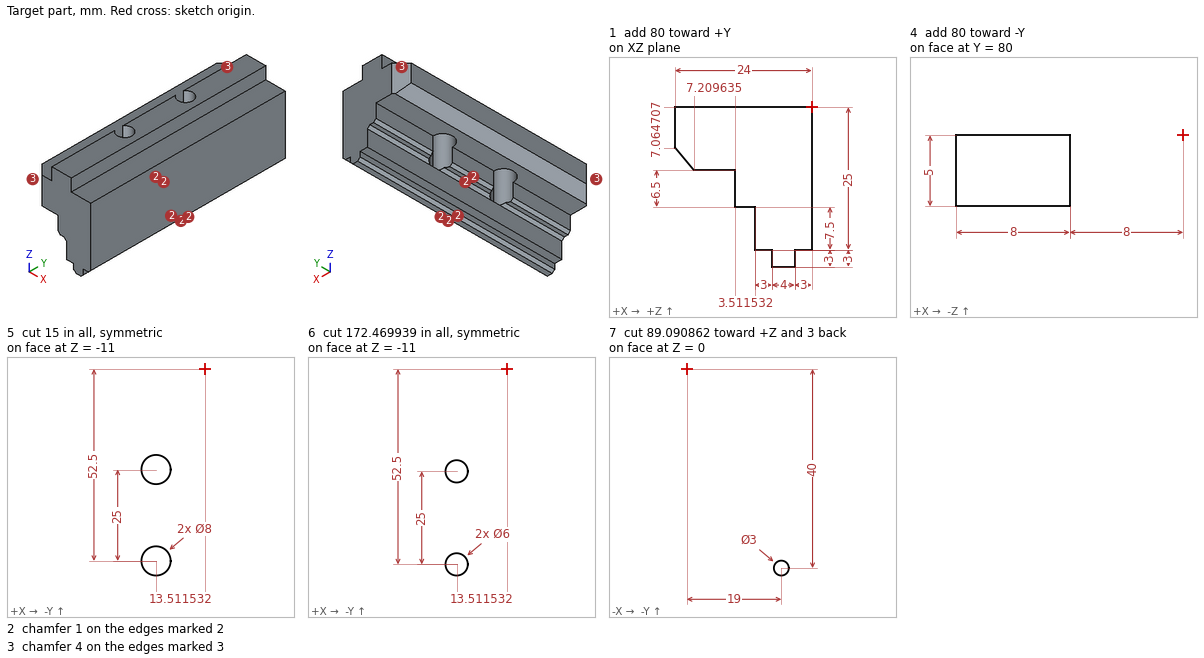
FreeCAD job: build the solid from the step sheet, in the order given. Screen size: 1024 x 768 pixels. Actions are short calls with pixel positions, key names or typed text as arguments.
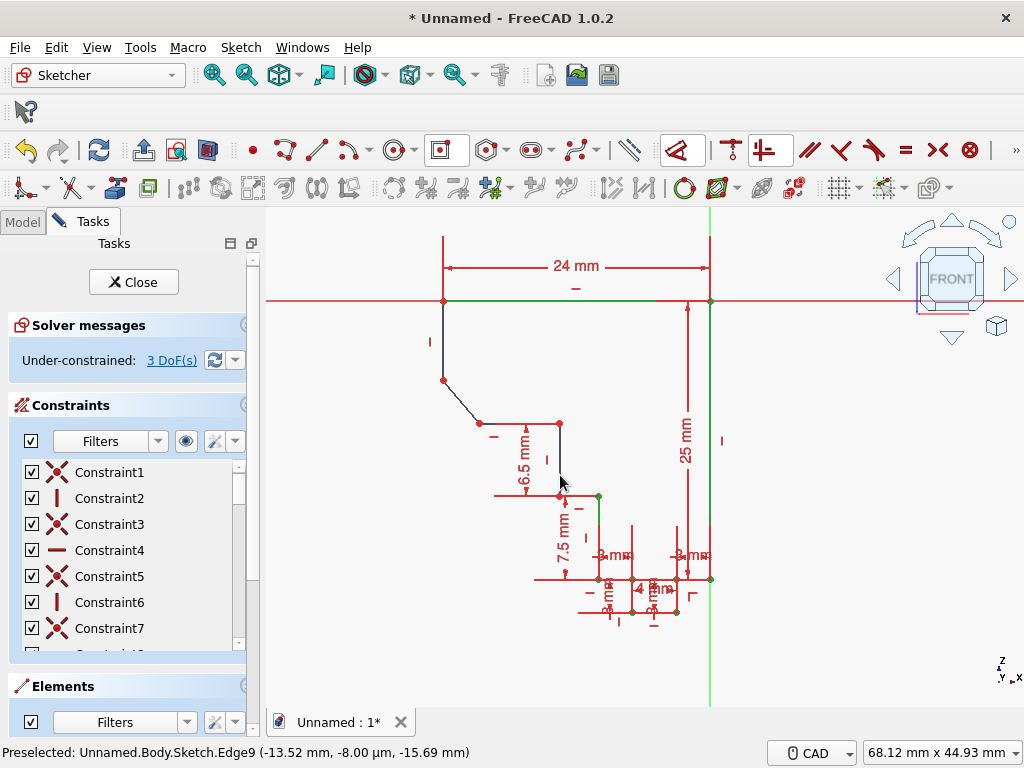
click(587, 496)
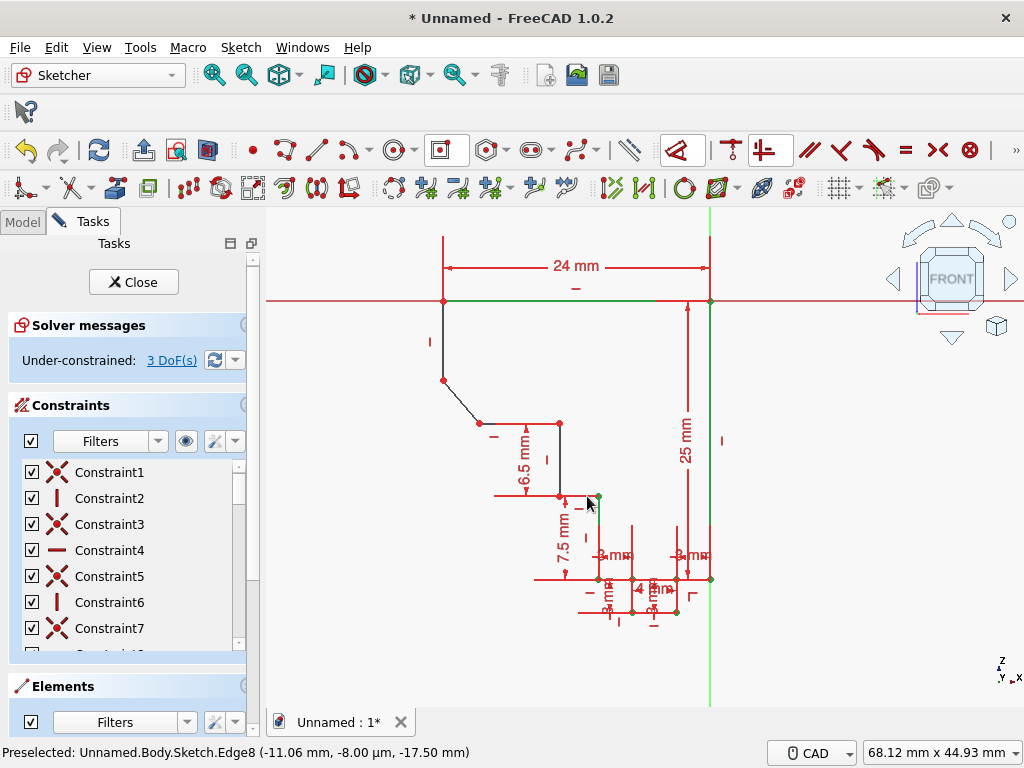
key(l)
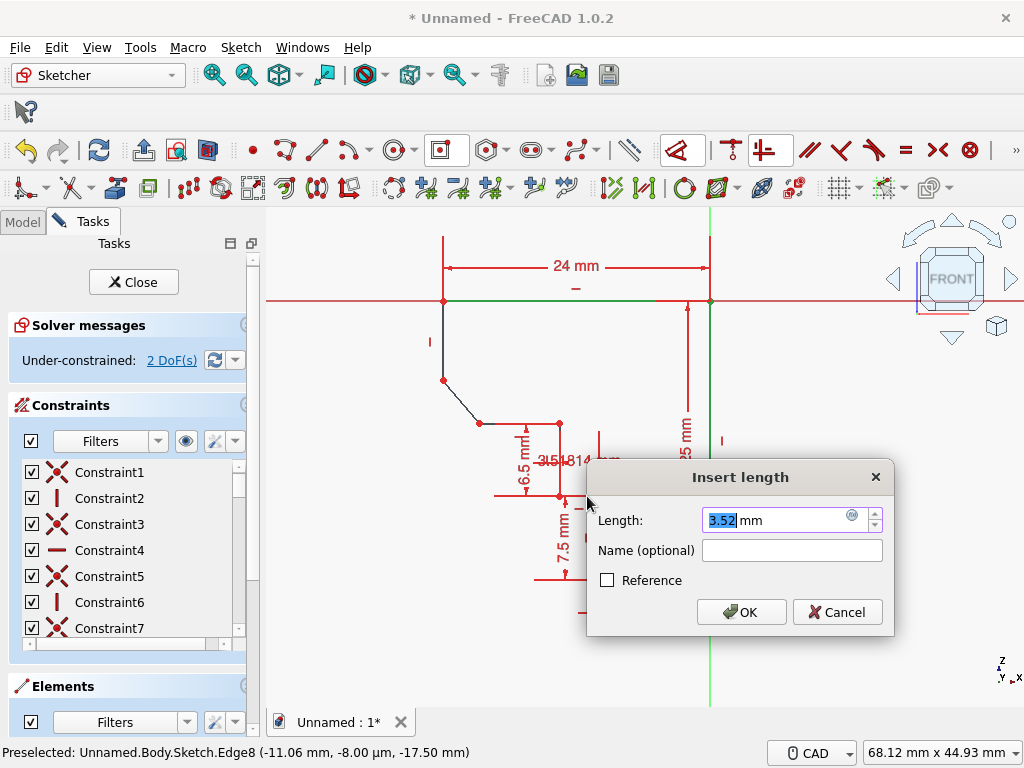
text(3.511532)
key(Return)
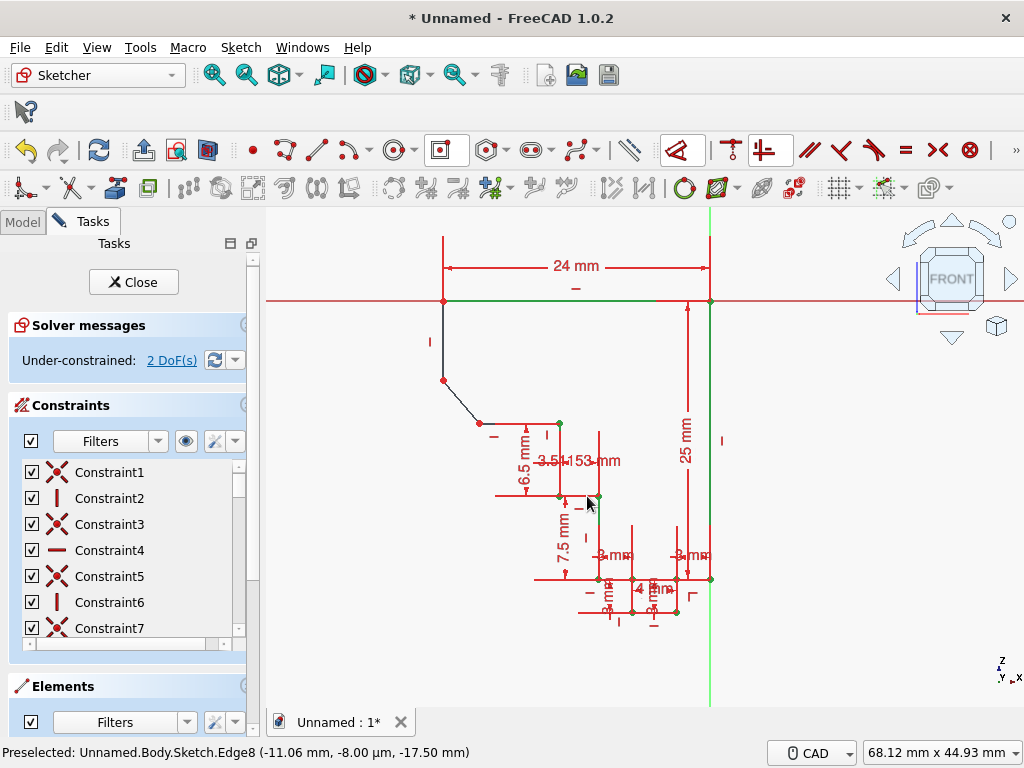
click(536, 424)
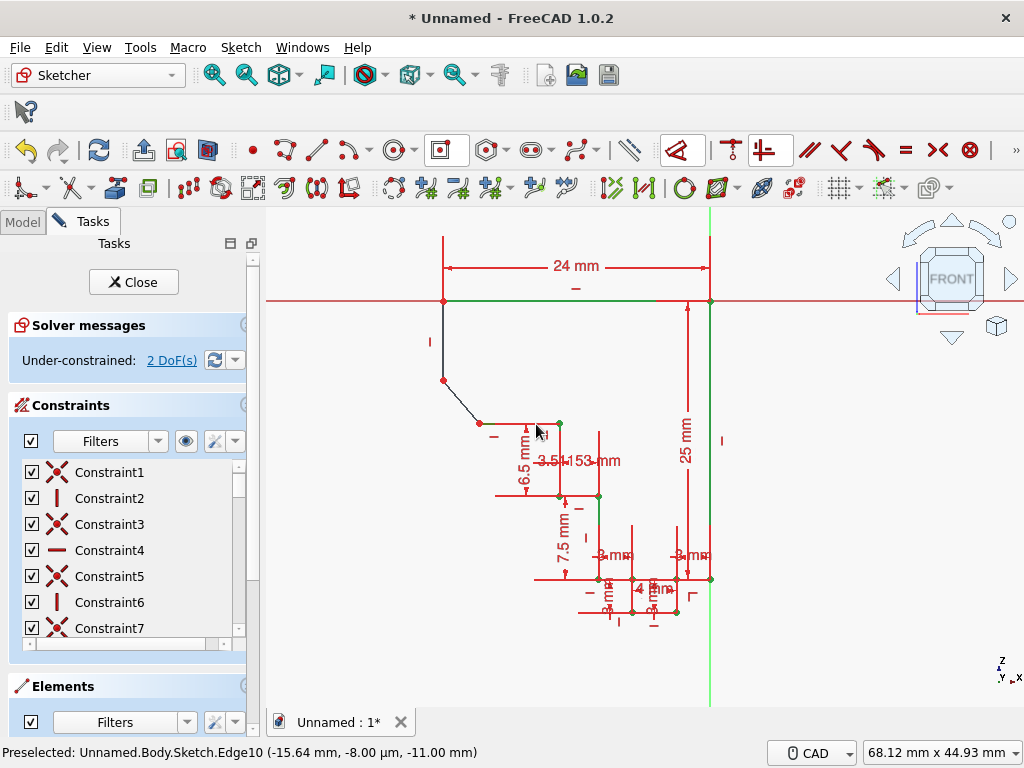
key(l)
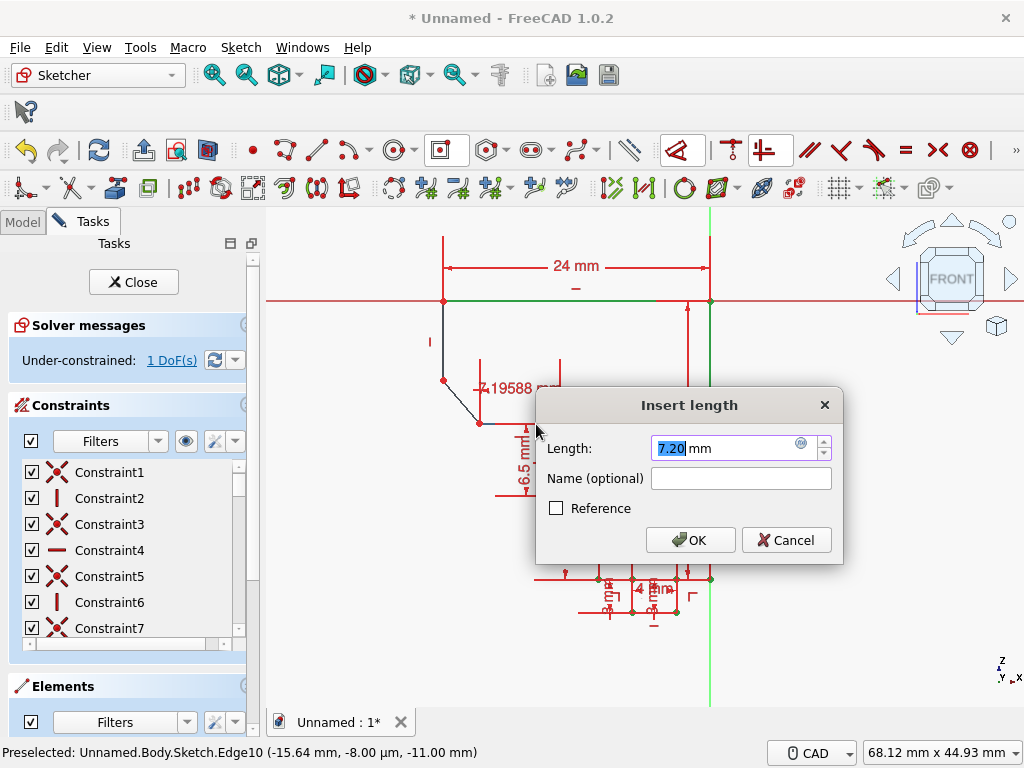
text(7.209635)
key(Return)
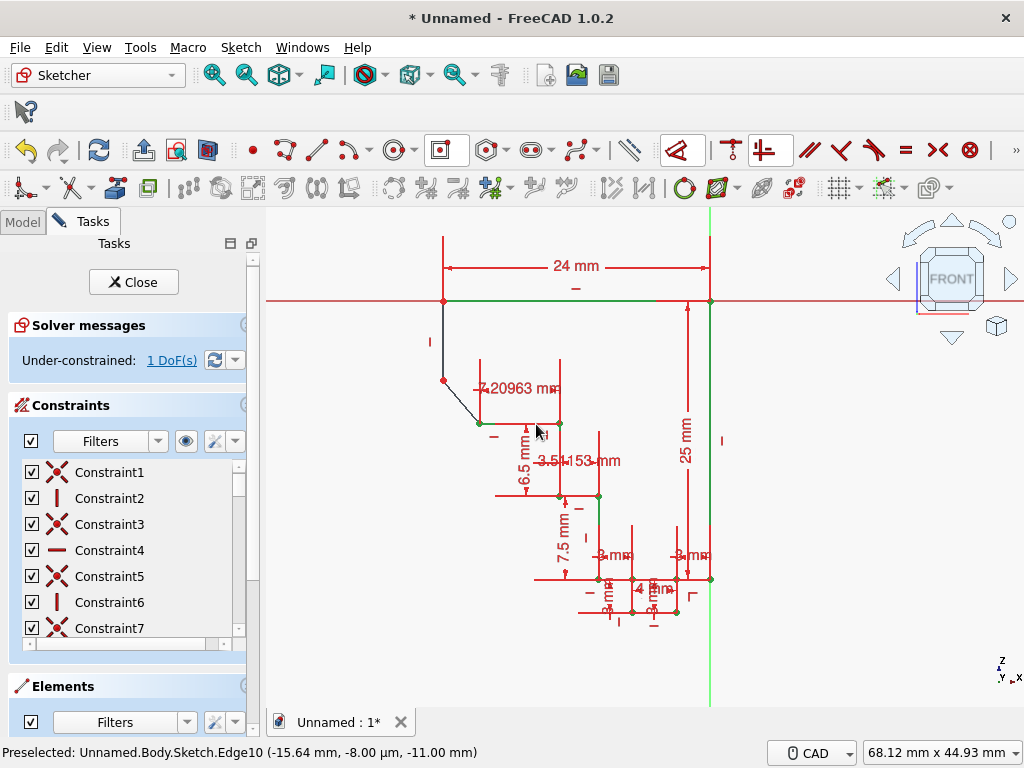
click(443, 357)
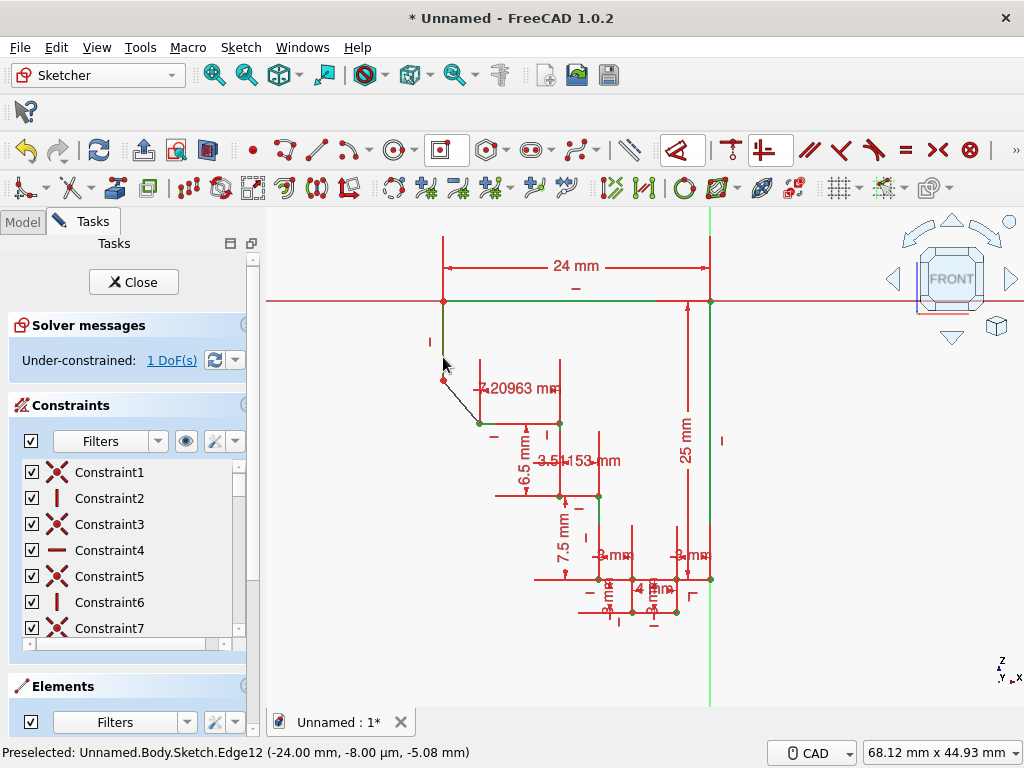
key(i)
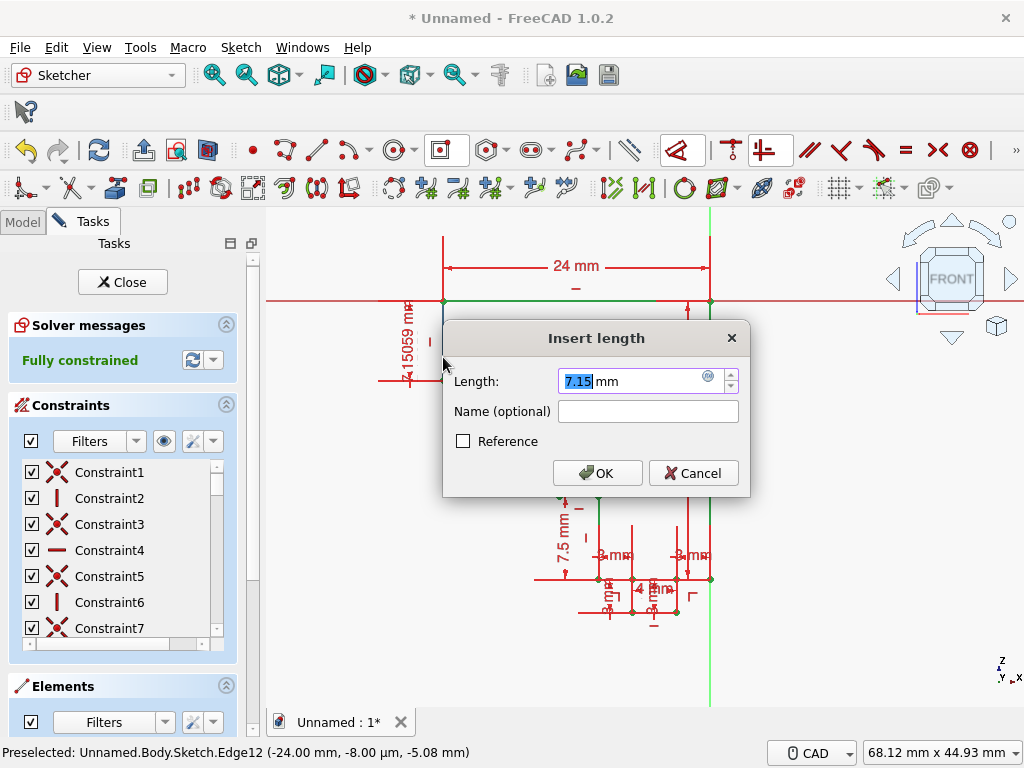
text(7.064707)
key(Return)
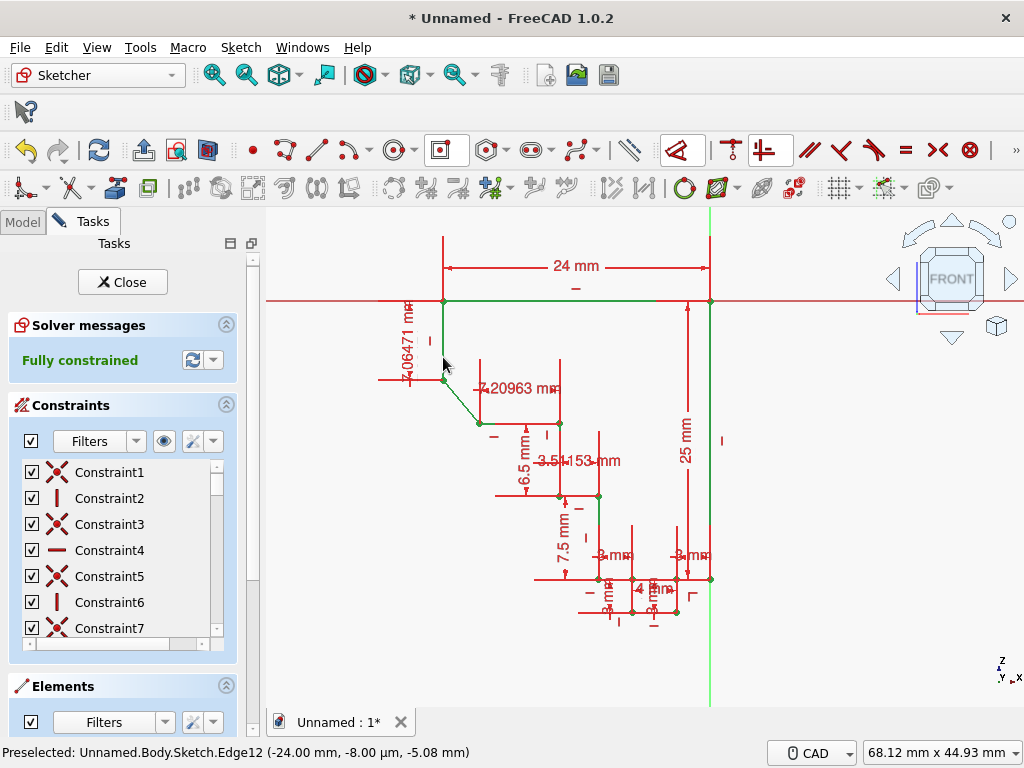
click(123, 282)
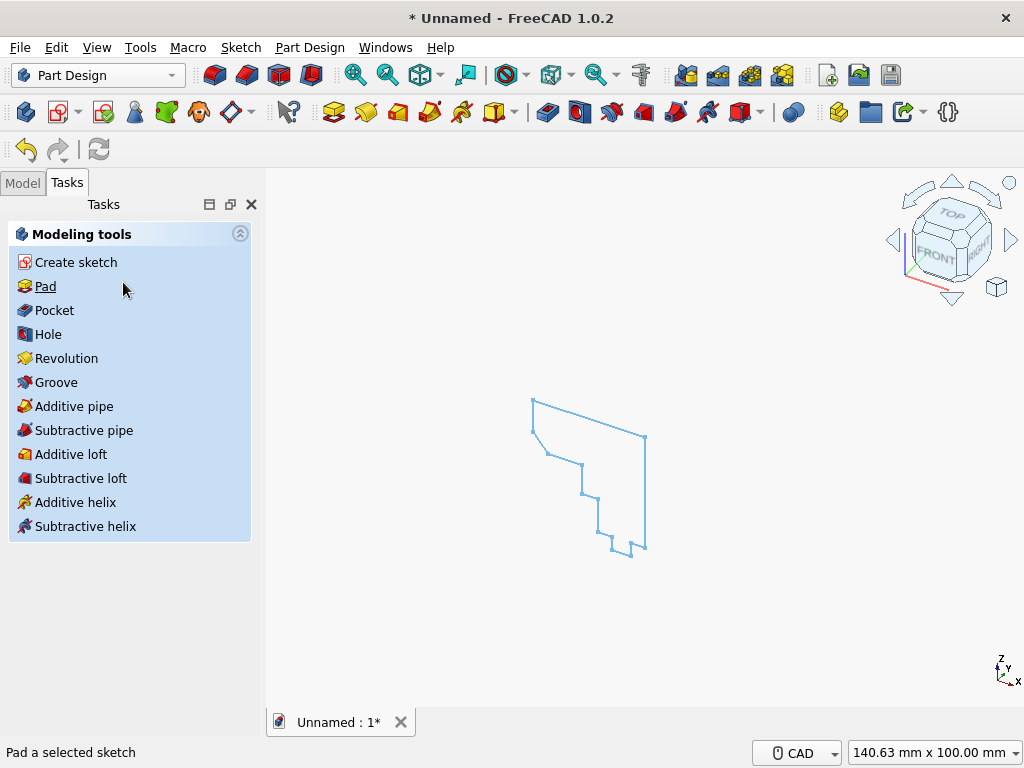
click(334, 112)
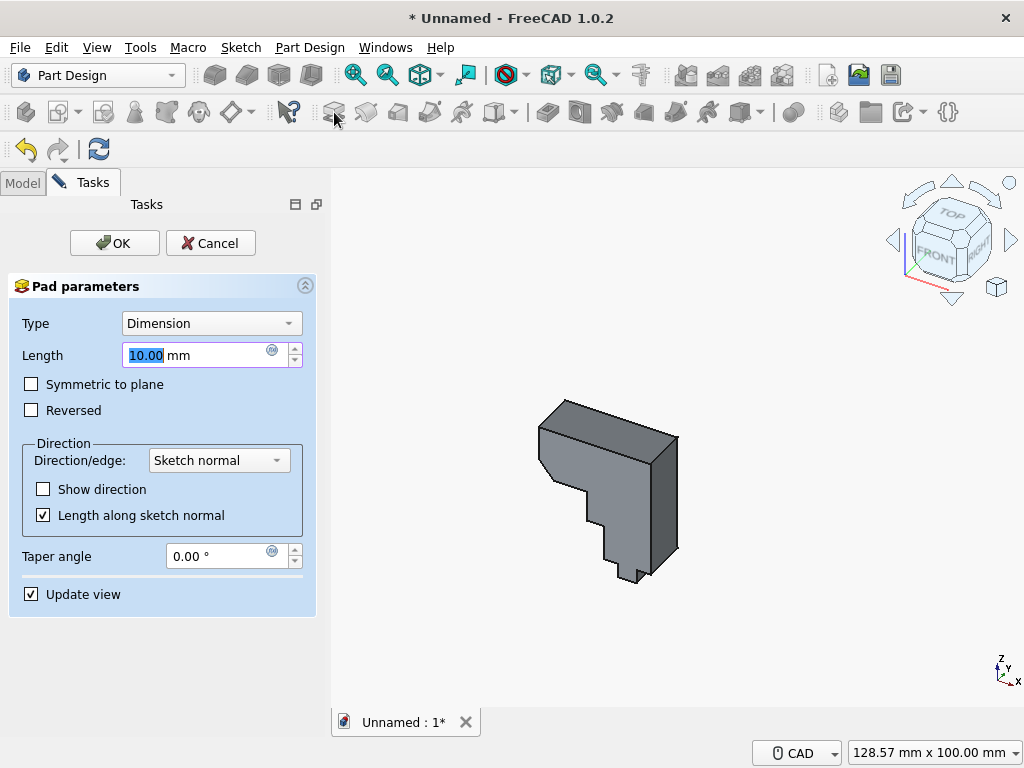
text(80)
key(Tab)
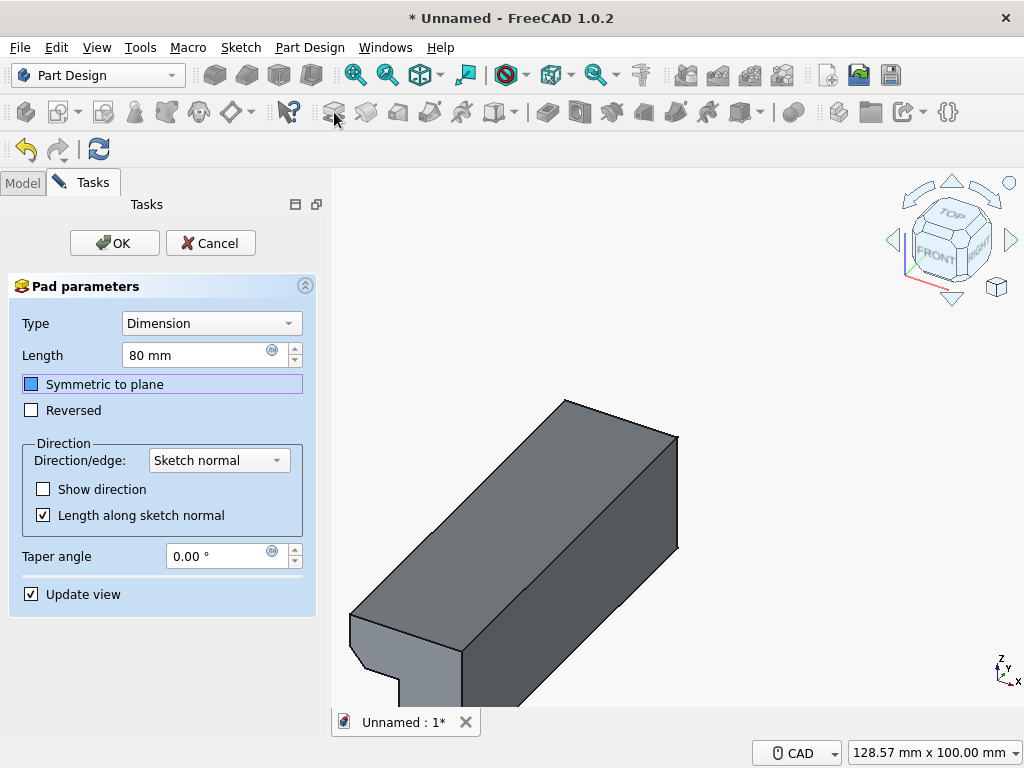
click(30, 410)